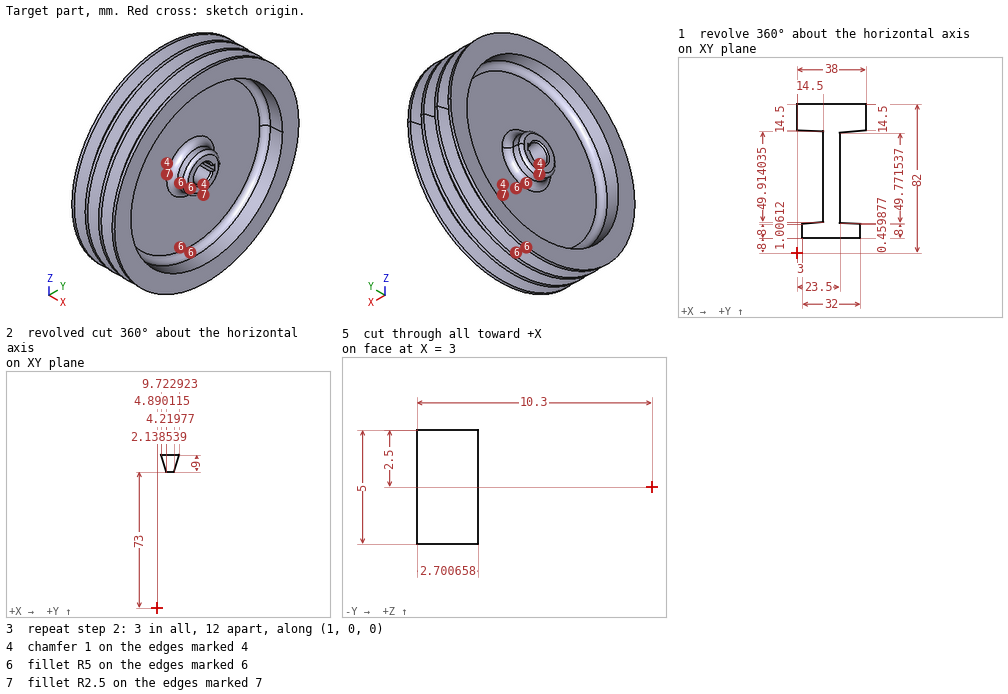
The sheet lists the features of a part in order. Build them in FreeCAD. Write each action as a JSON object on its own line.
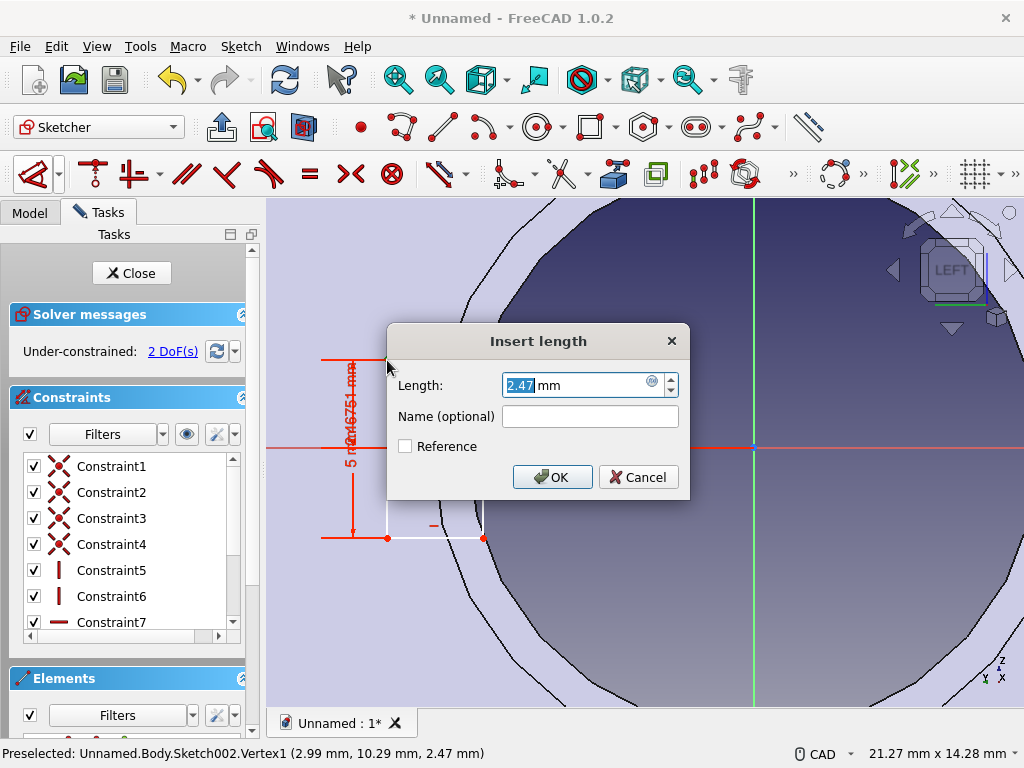
{"action": "type", "text": "2.5"}
{"action": "key", "text": "Return"}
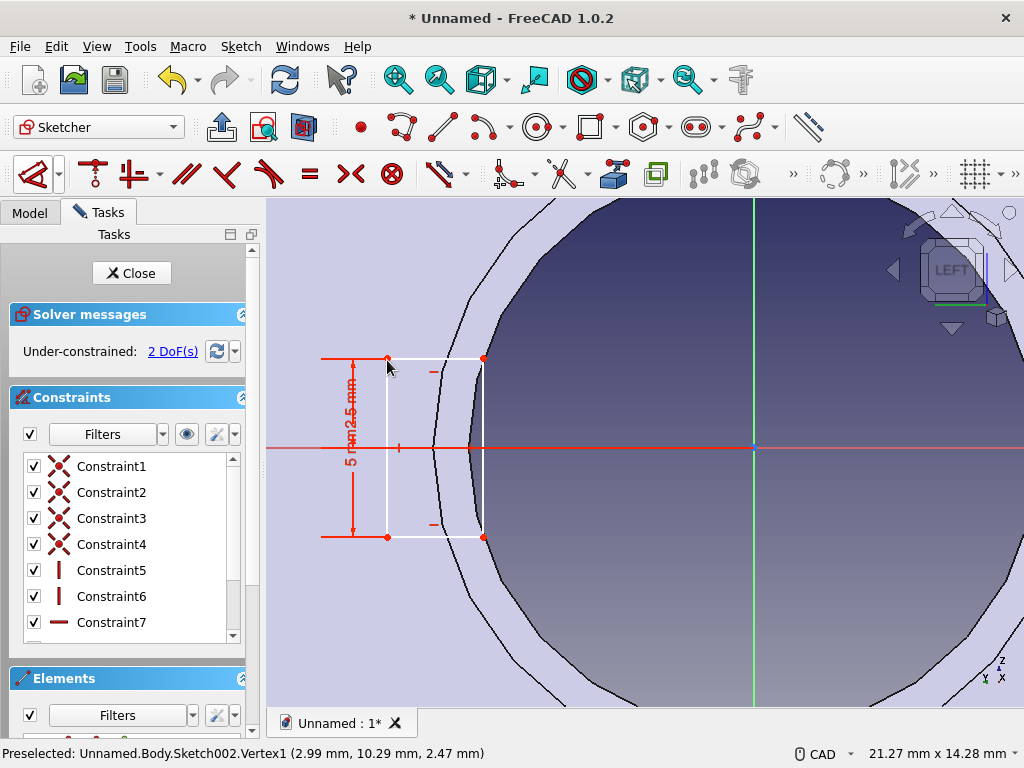
{"action": "left_click", "coordinate": [387, 359]}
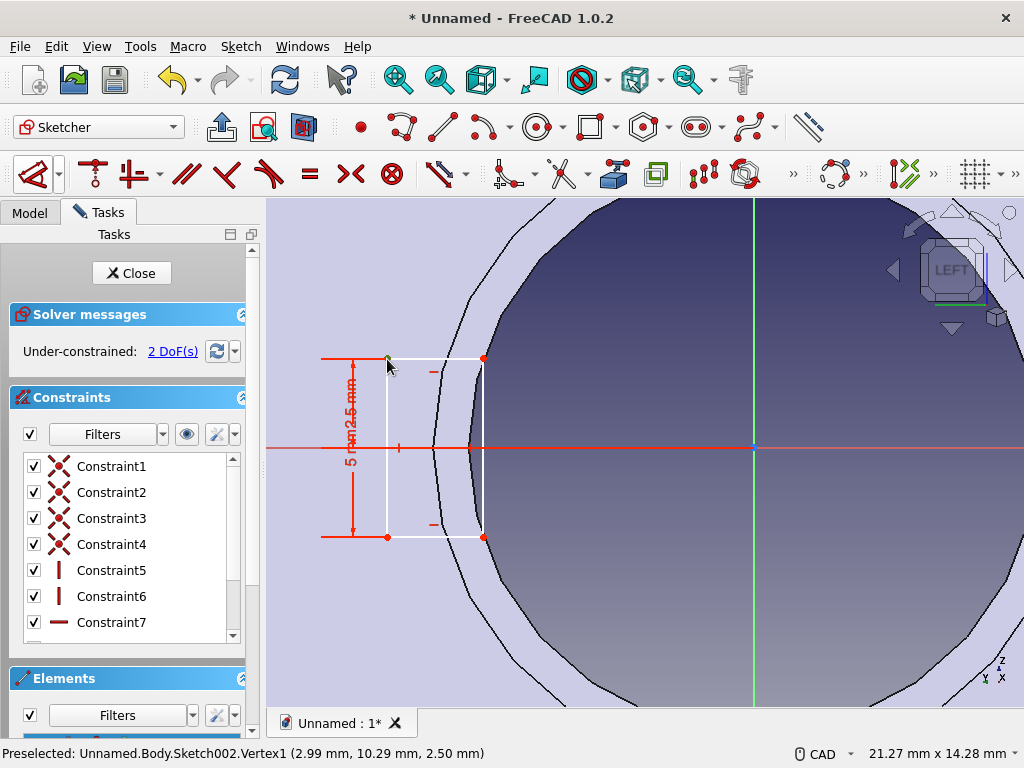
{"action": "left_click", "coordinate": [58, 174]}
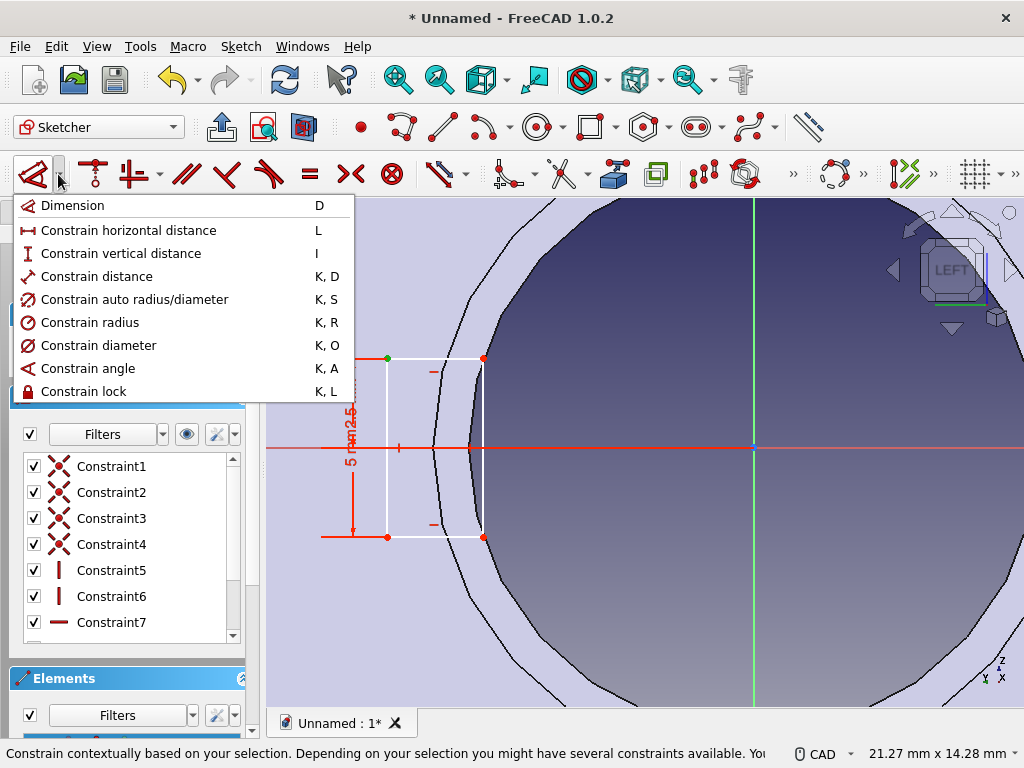
{"action": "left_click", "coordinate": [184, 230]}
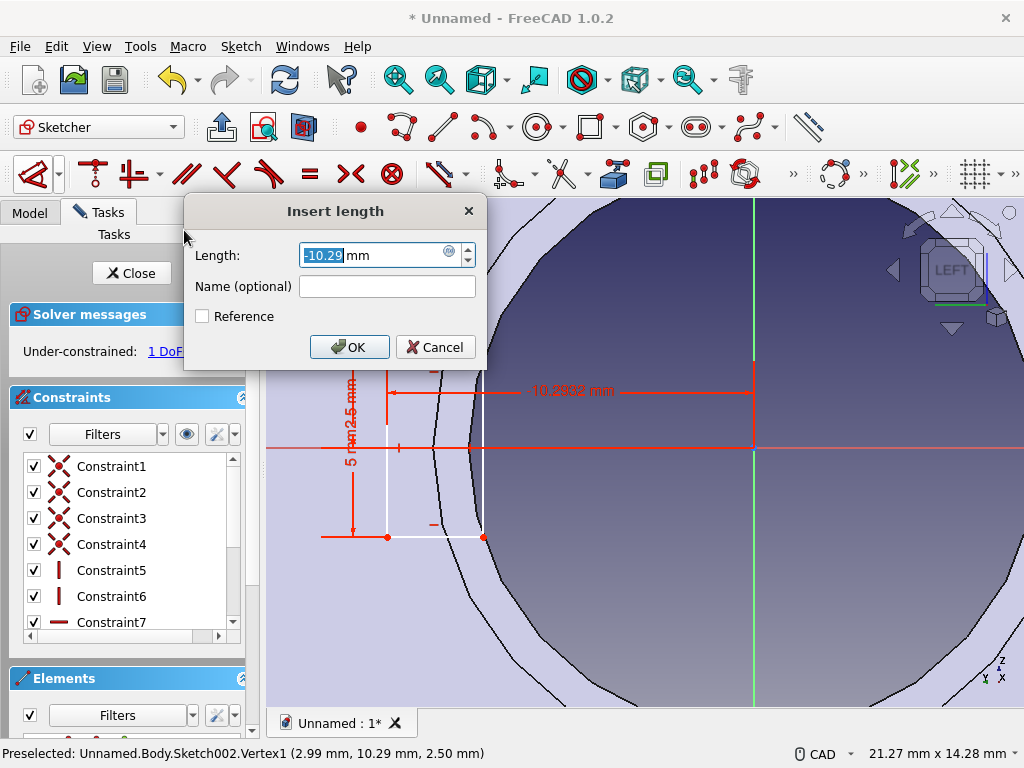
{"action": "type", "text": "-10.3"}
{"action": "key", "text": "Return"}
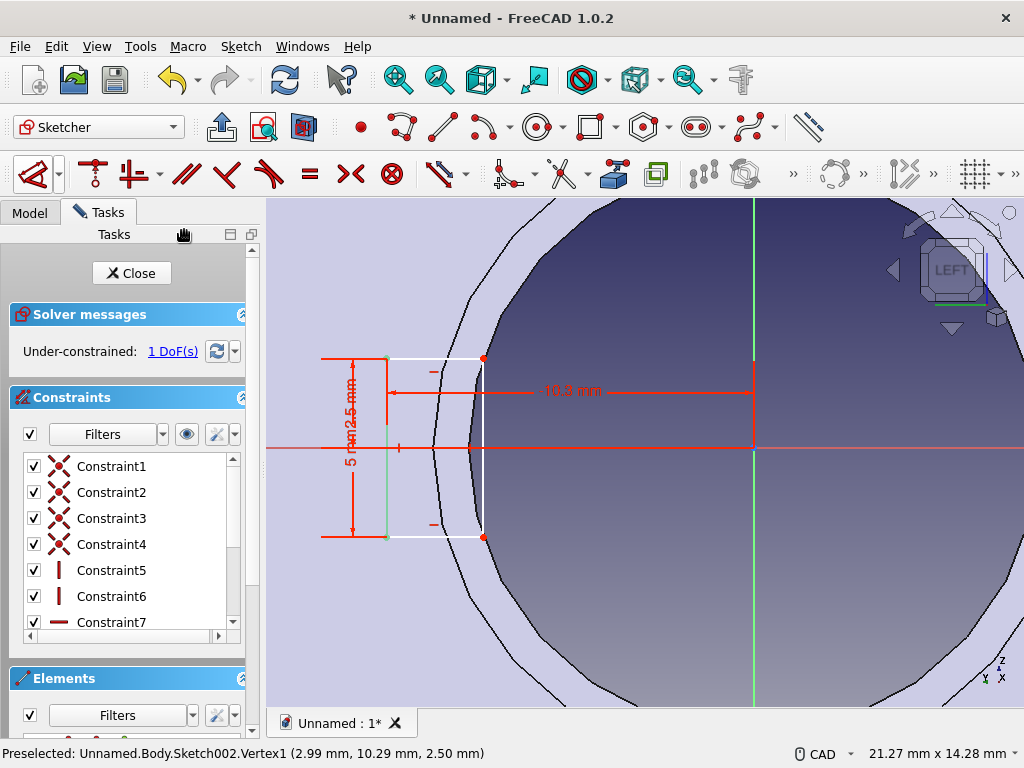
{"action": "left_click", "coordinate": [416, 537]}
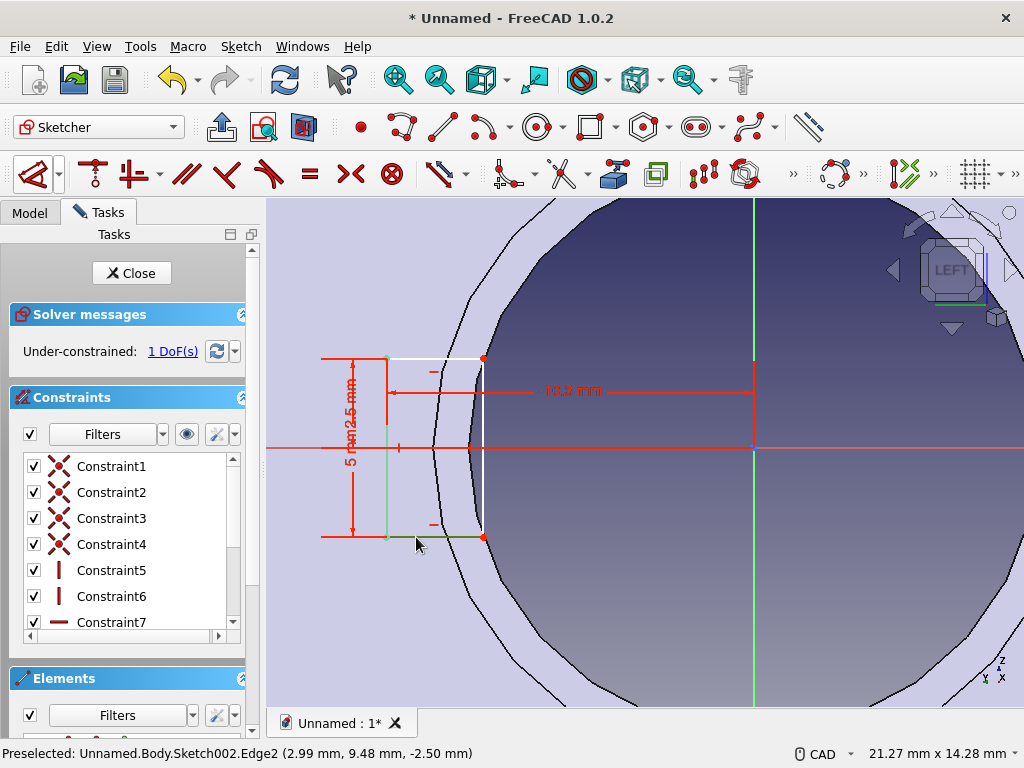
{"action": "left_click", "coordinate": [58, 174]}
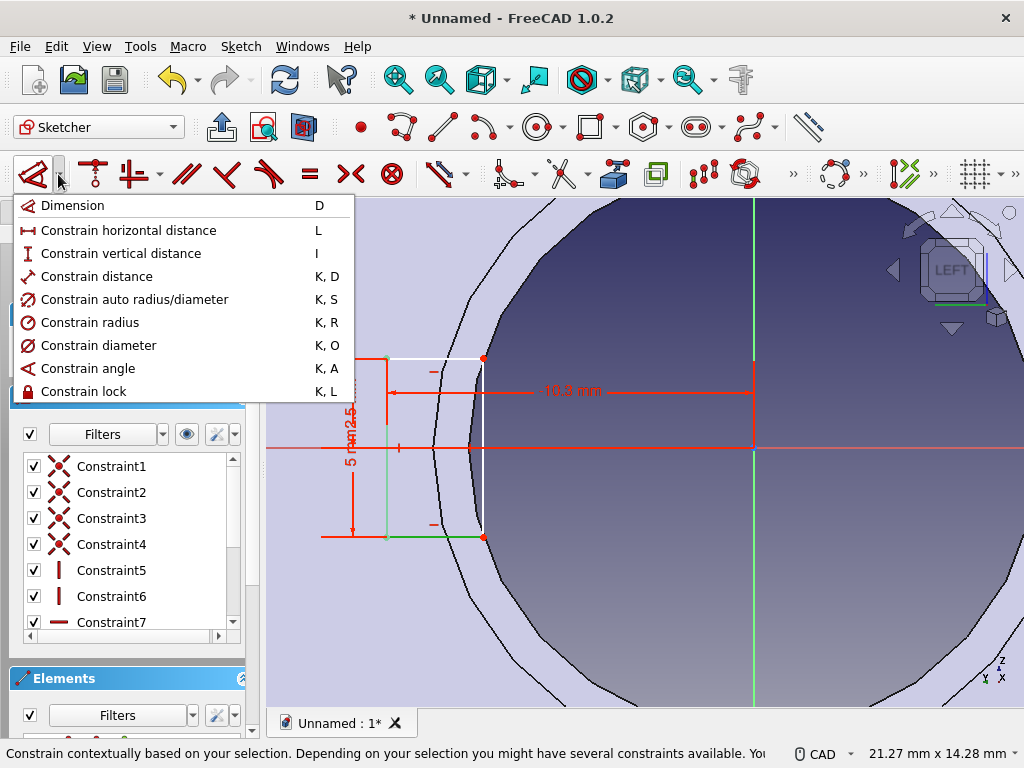
{"action": "left_click", "coordinate": [184, 230]}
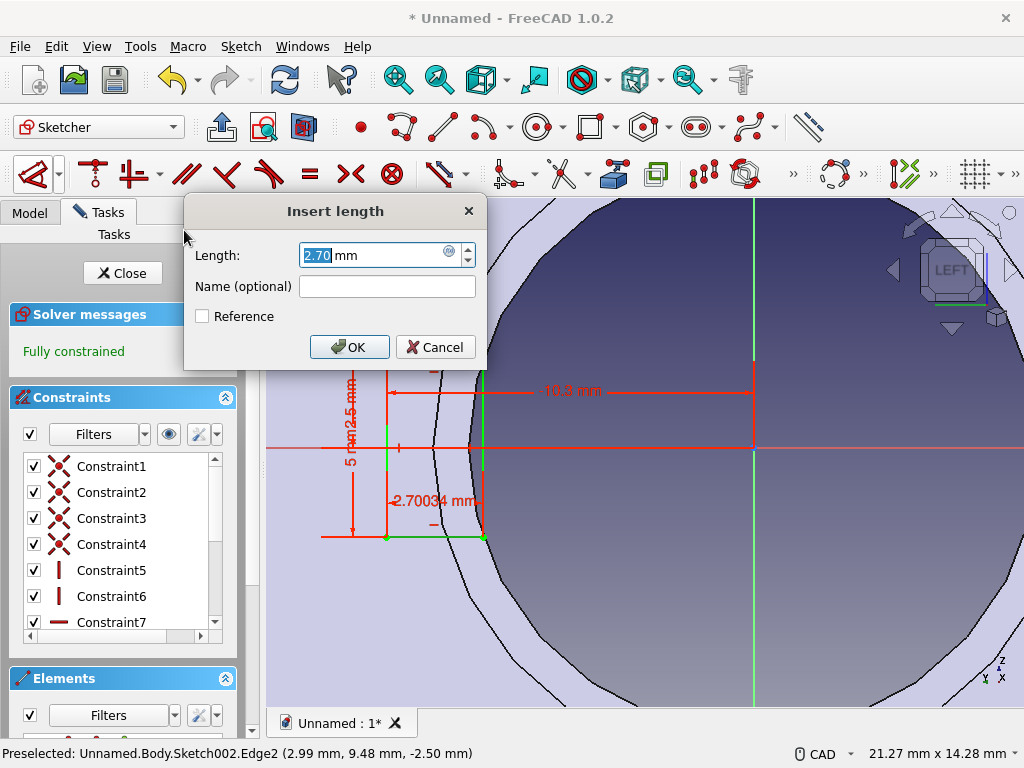
{"action": "type", "text": "2.700658"}
{"action": "key", "text": "Return"}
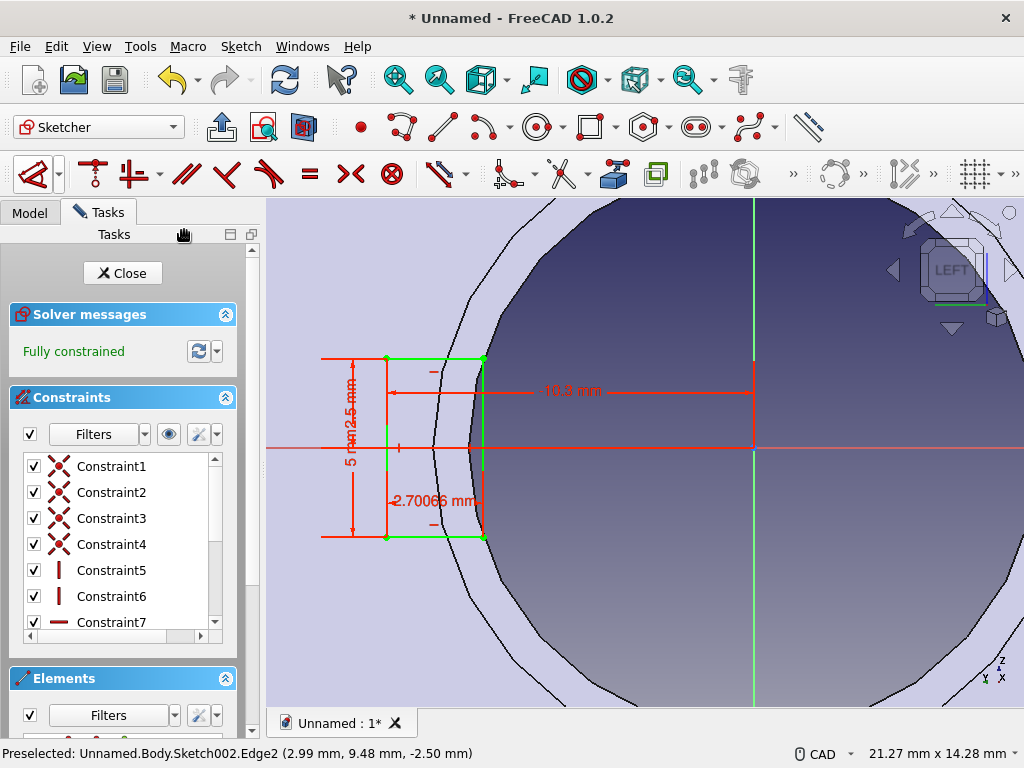
{"action": "left_click", "coordinate": [123, 273]}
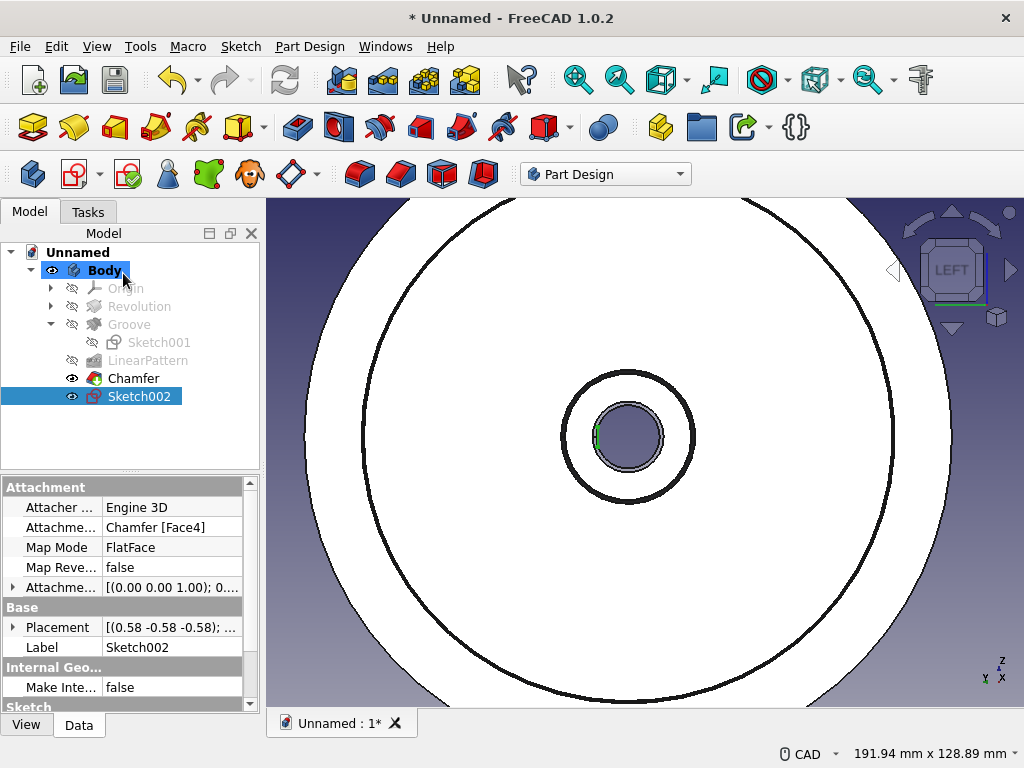
{"action": "left_click", "coordinate": [298, 128]}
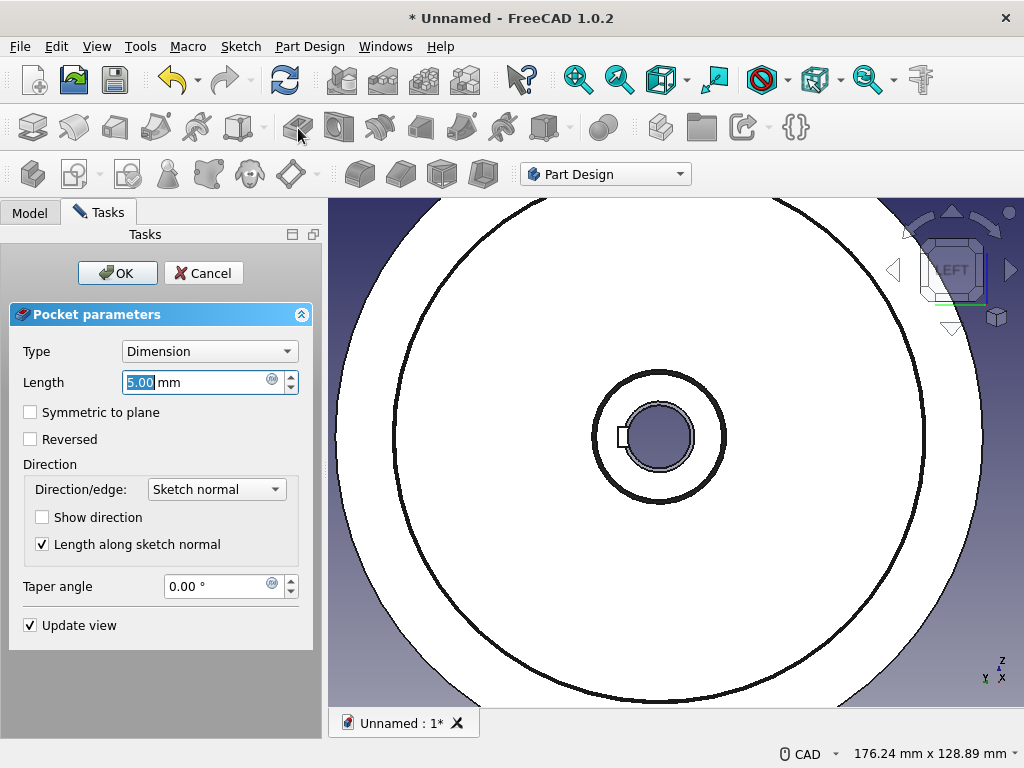
{"action": "left_click", "coordinate": [210, 352]}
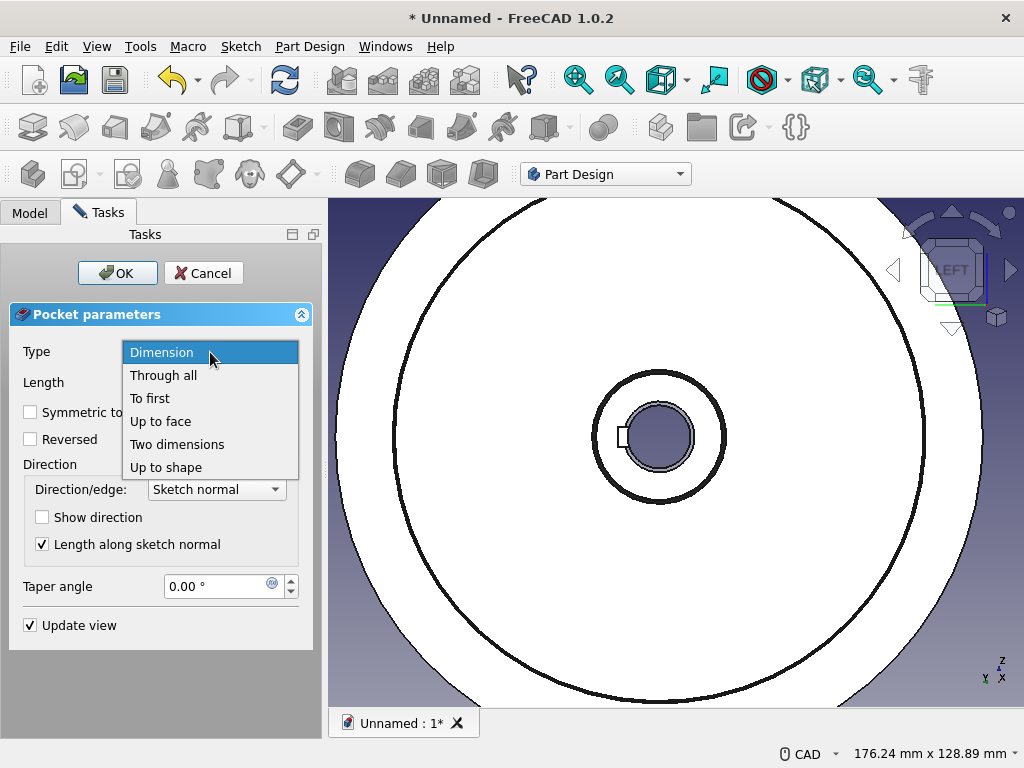
{"action": "left_click", "coordinate": [208, 376]}